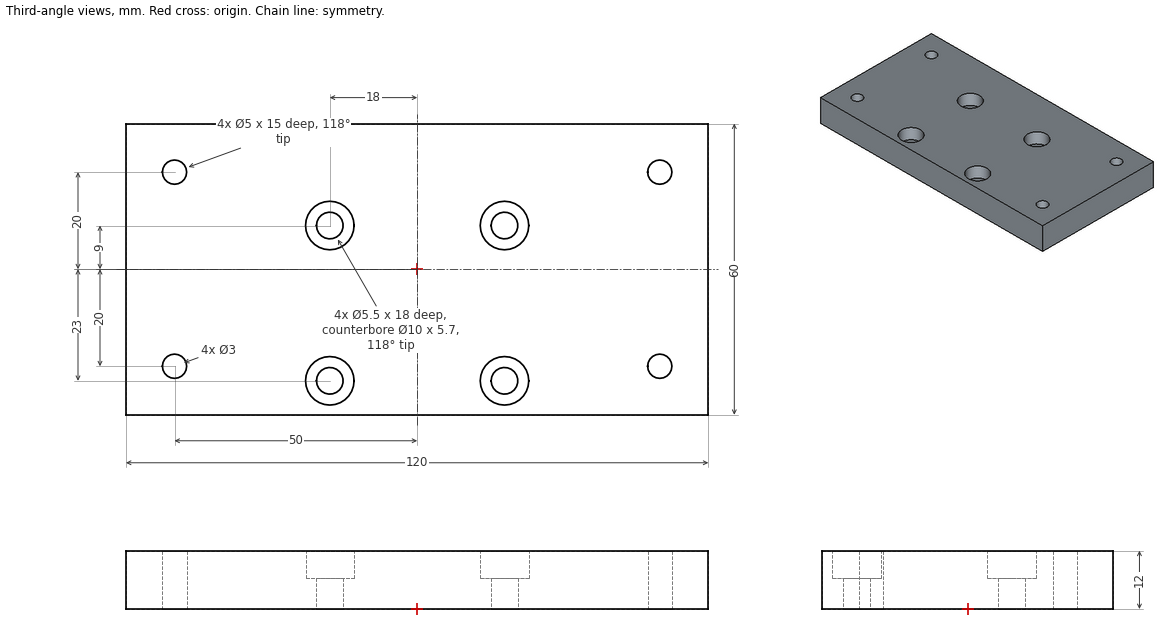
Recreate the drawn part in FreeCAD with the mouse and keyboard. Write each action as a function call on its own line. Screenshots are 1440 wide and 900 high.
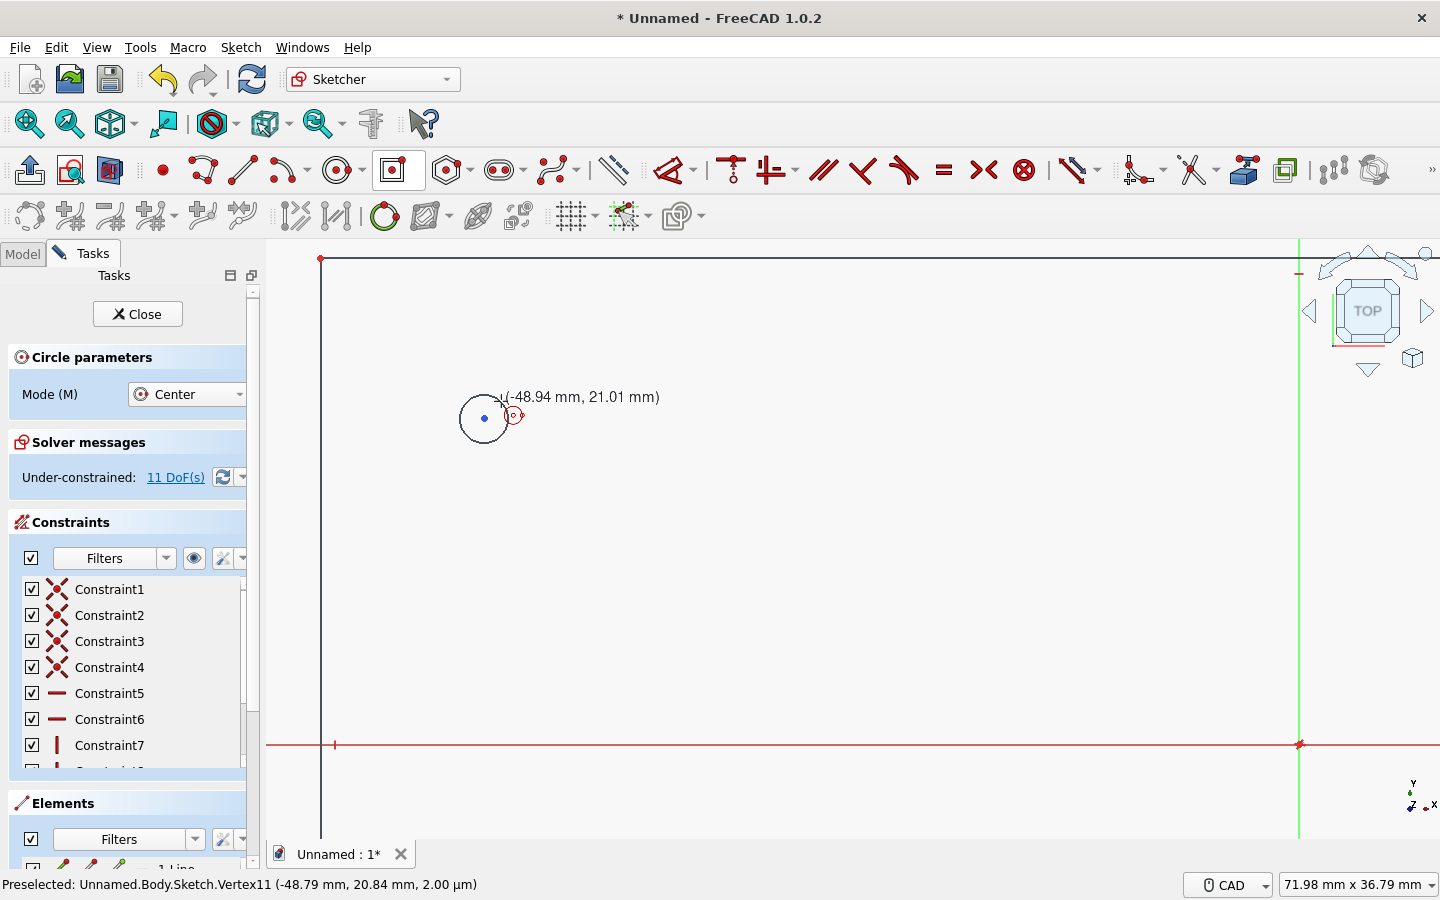
scroll(485, 419, down, 5)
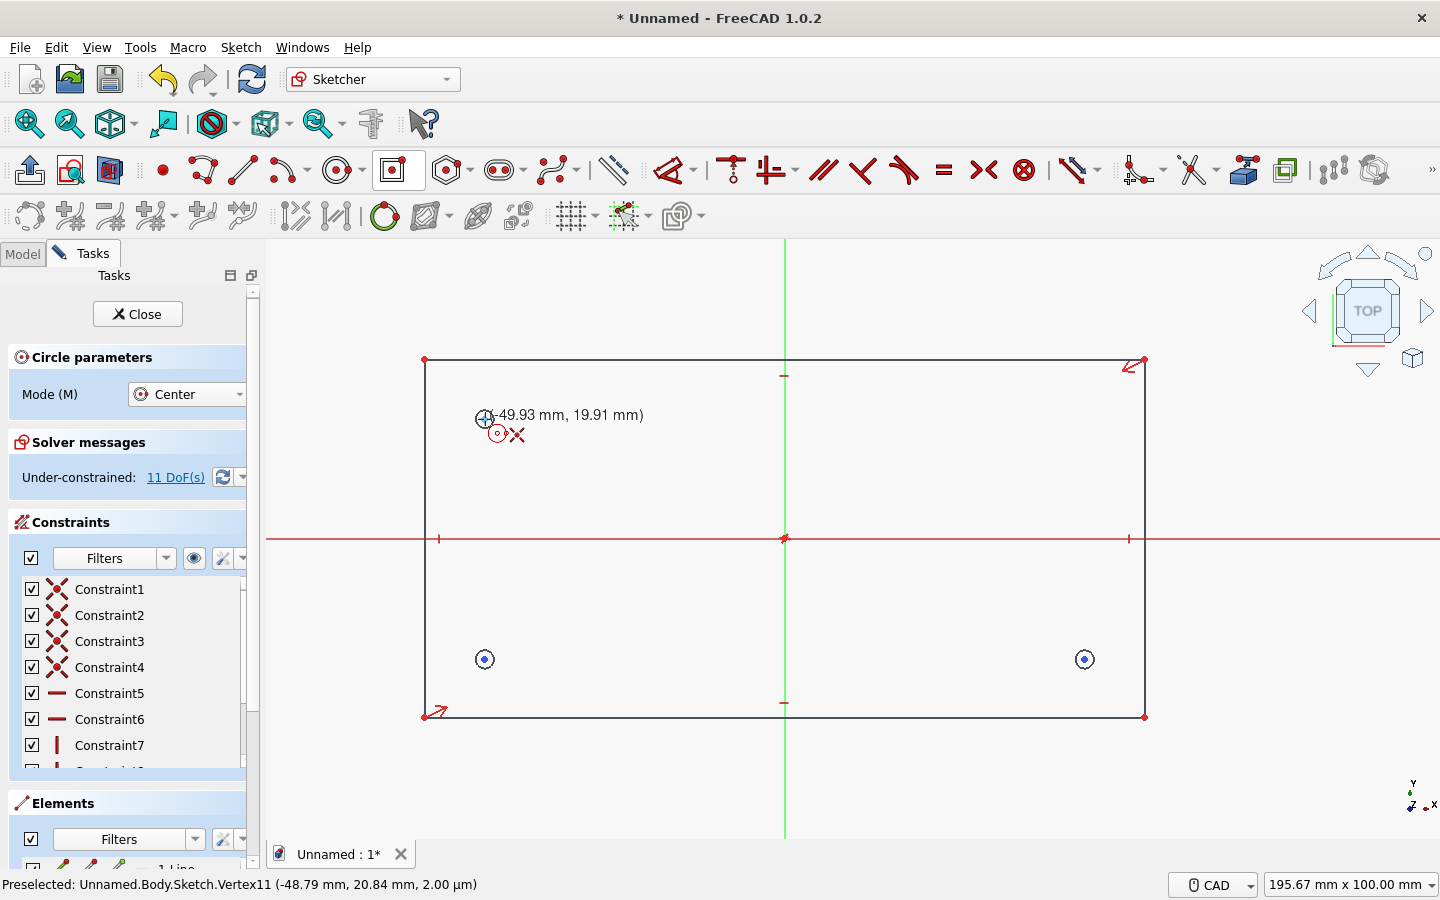
scroll(1085, 419, up, 5)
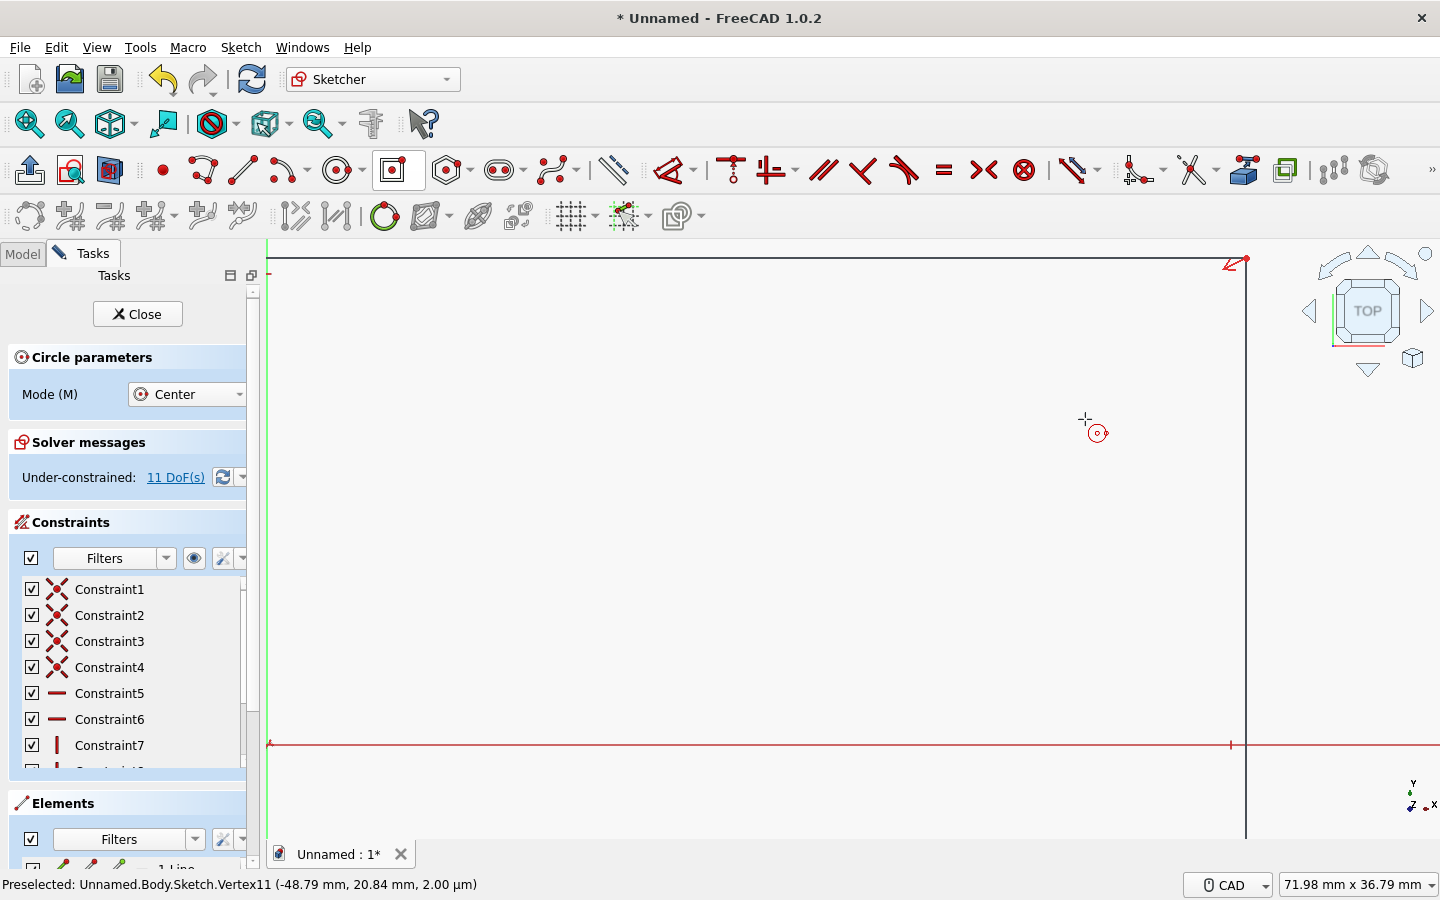
click(1083, 418)
click(1100, 401)
key(Escape)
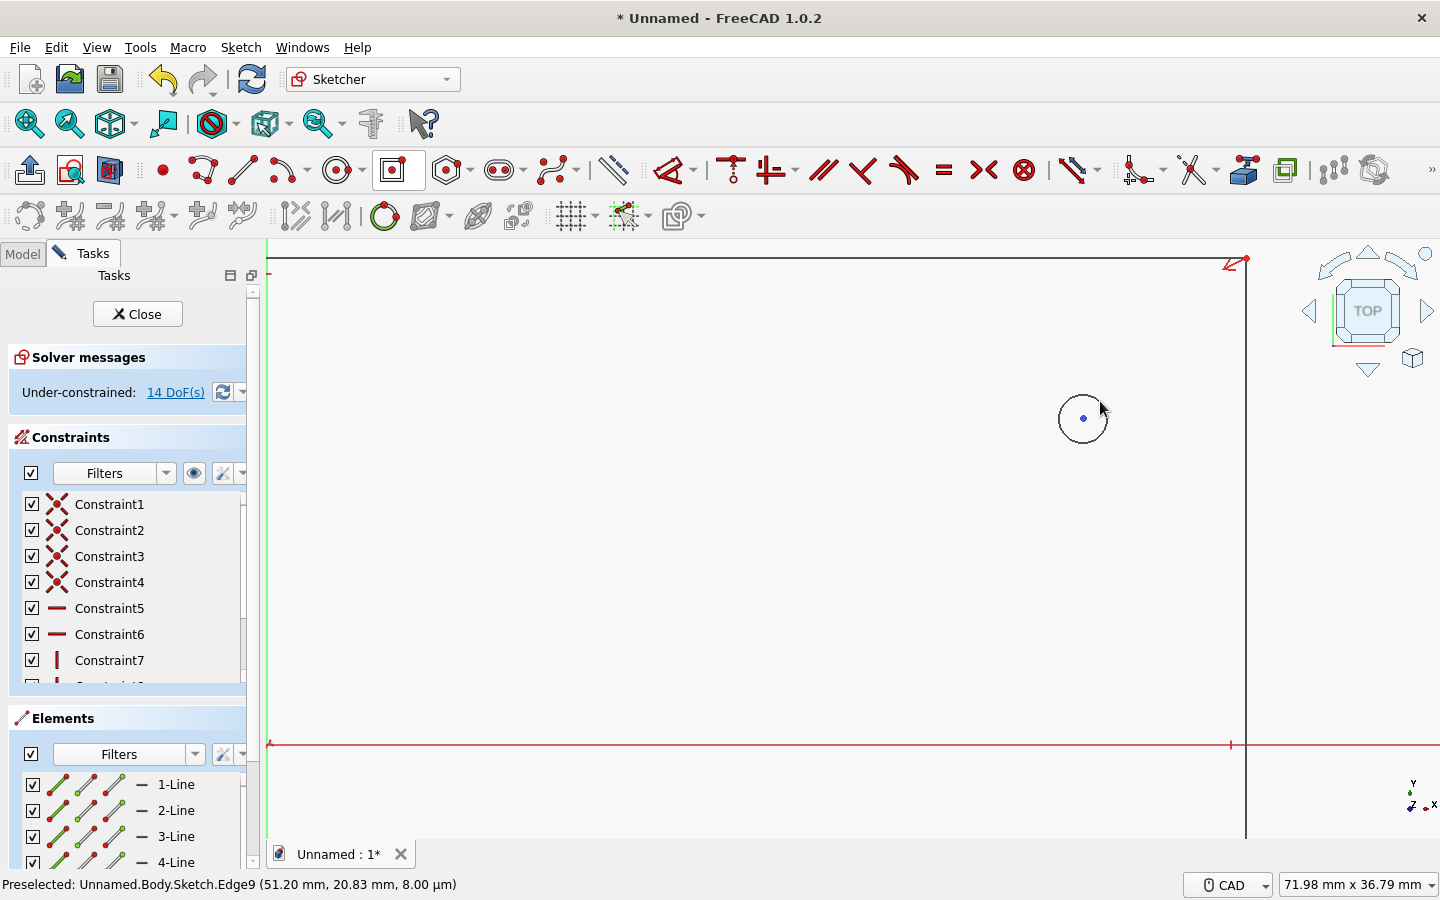
scroll(1085, 419, down, 5)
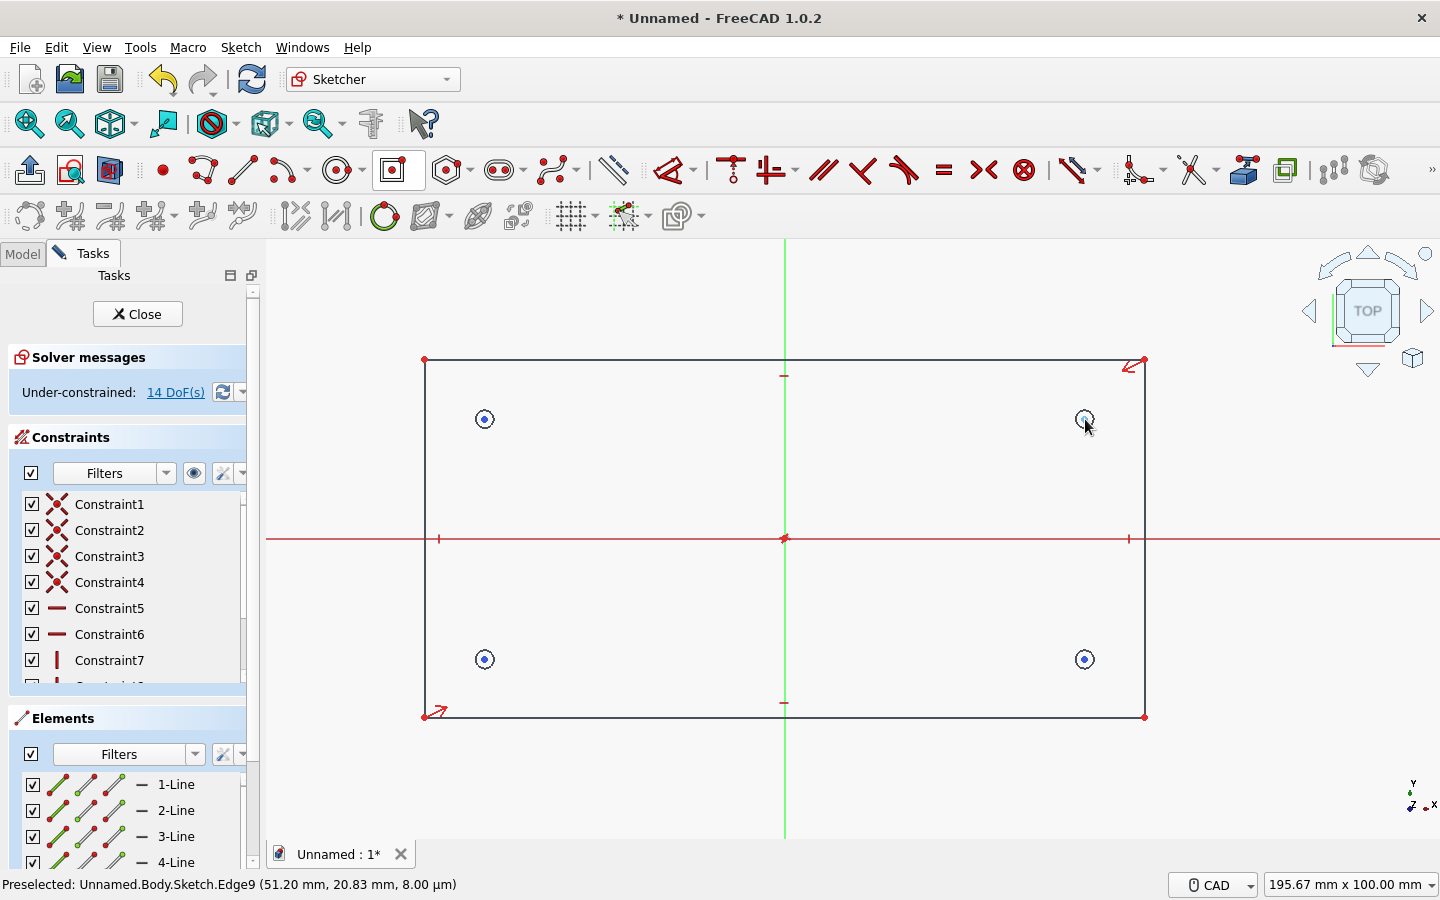
scroll(491, 653, up, 3)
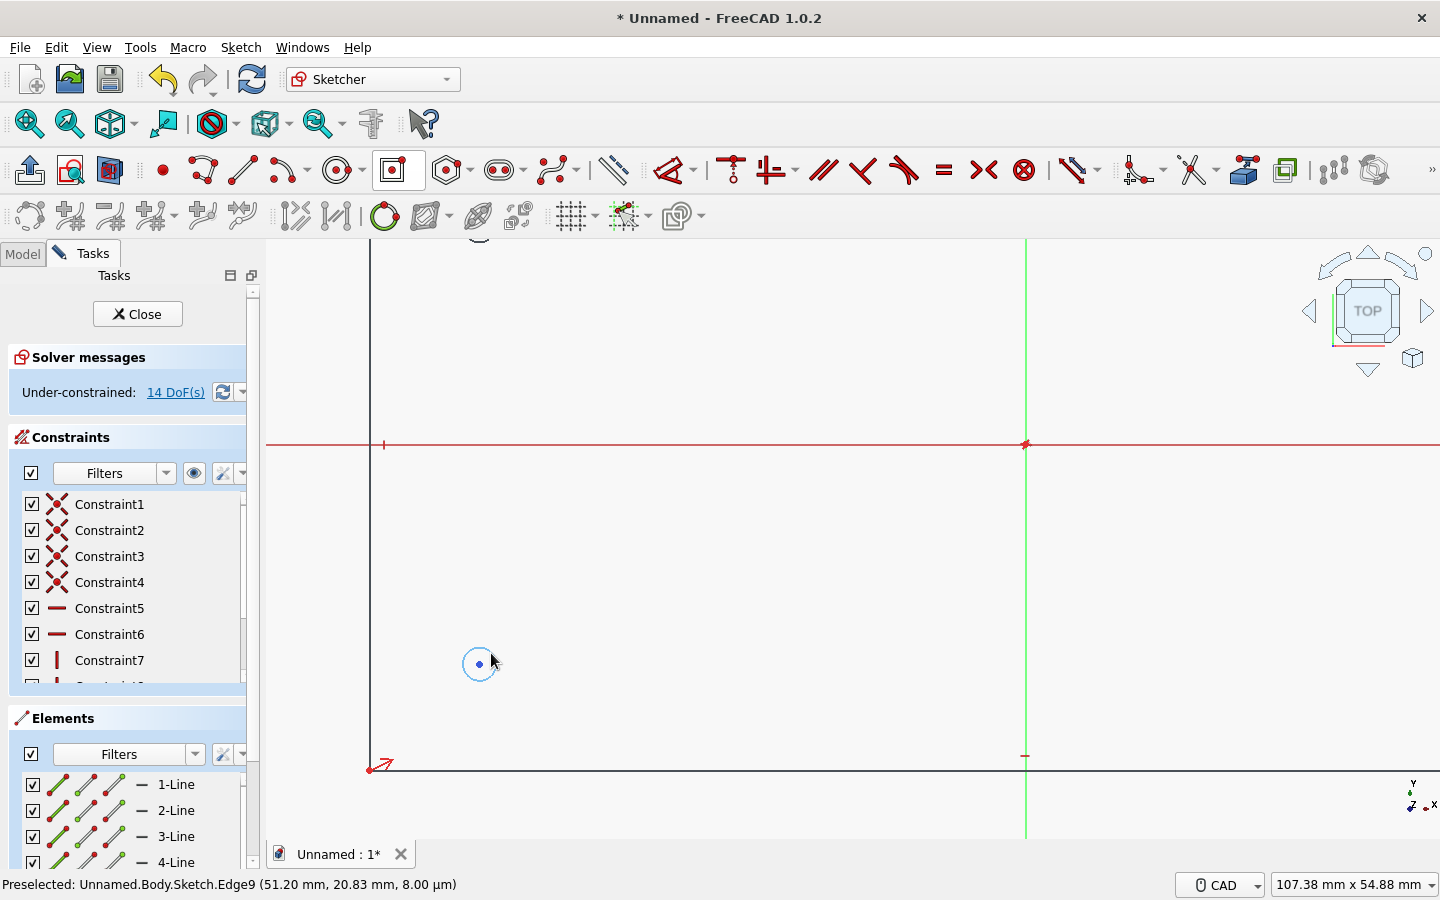
click(491, 652)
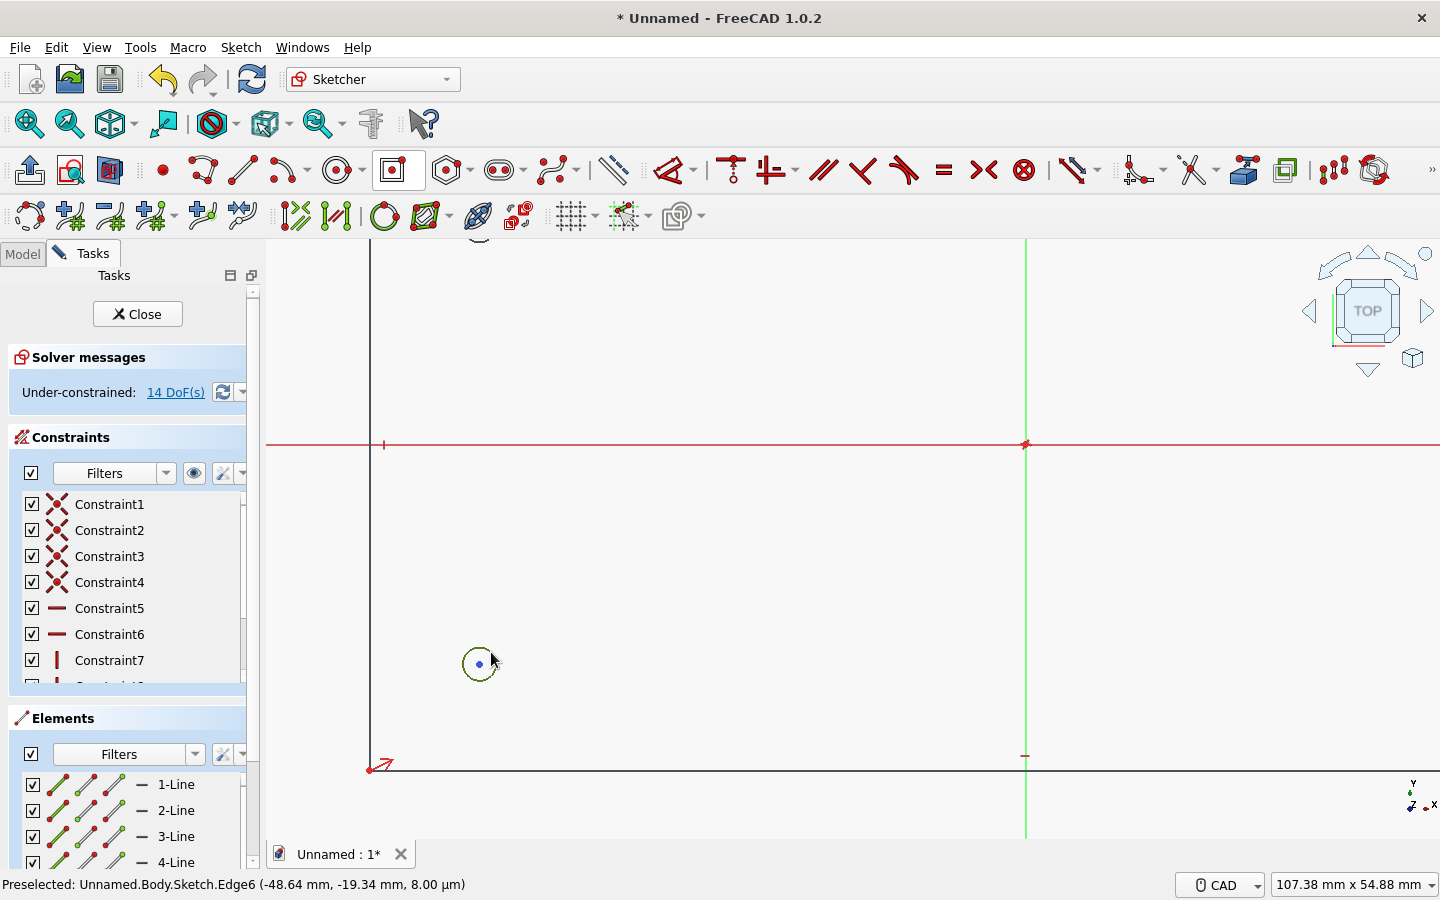
scroll(491, 654, down, 3)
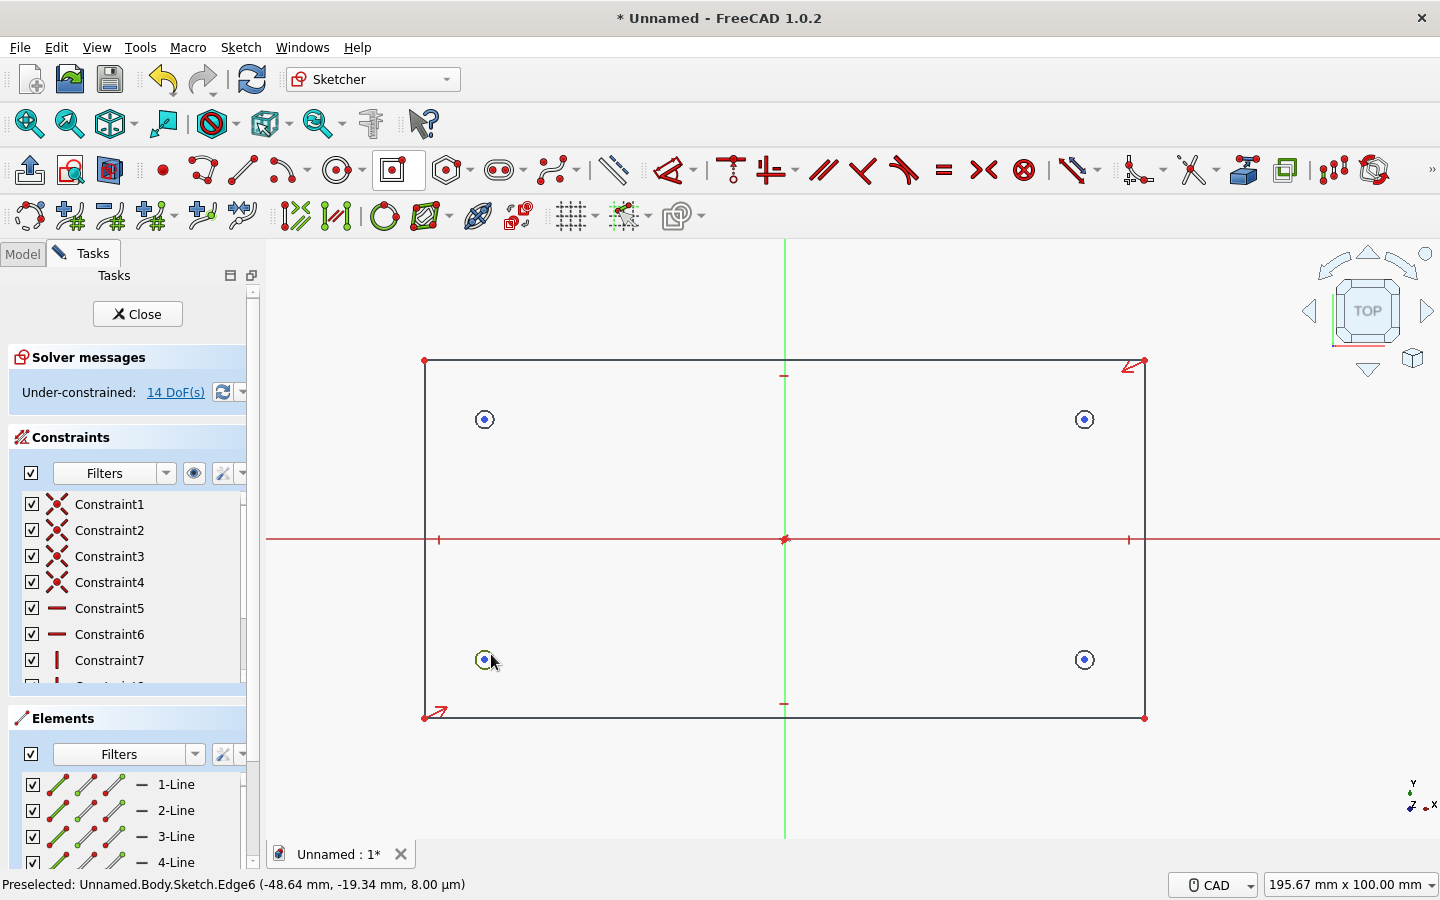
scroll(1091, 653, up, 3)